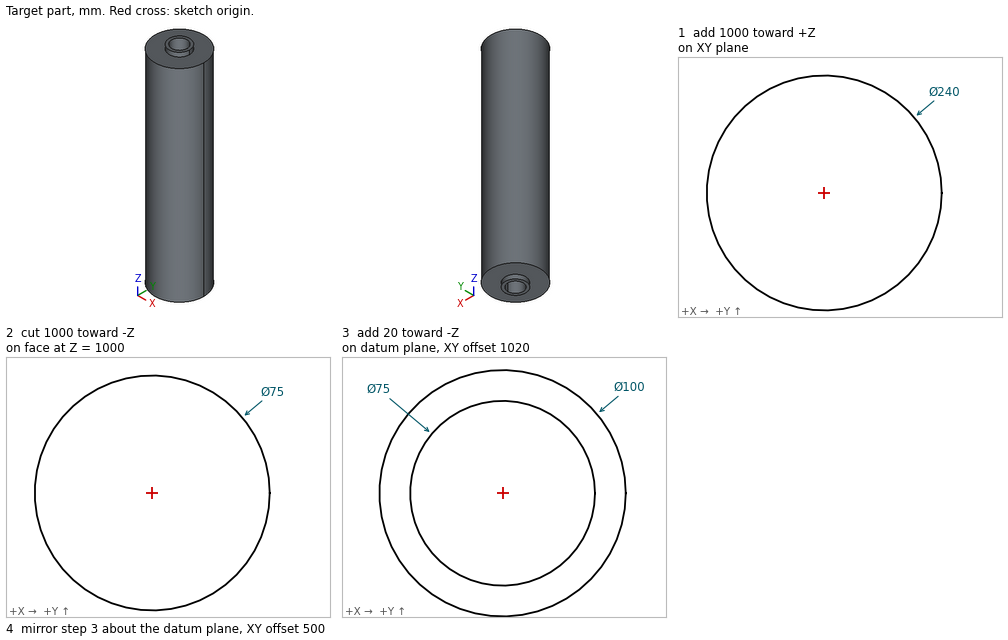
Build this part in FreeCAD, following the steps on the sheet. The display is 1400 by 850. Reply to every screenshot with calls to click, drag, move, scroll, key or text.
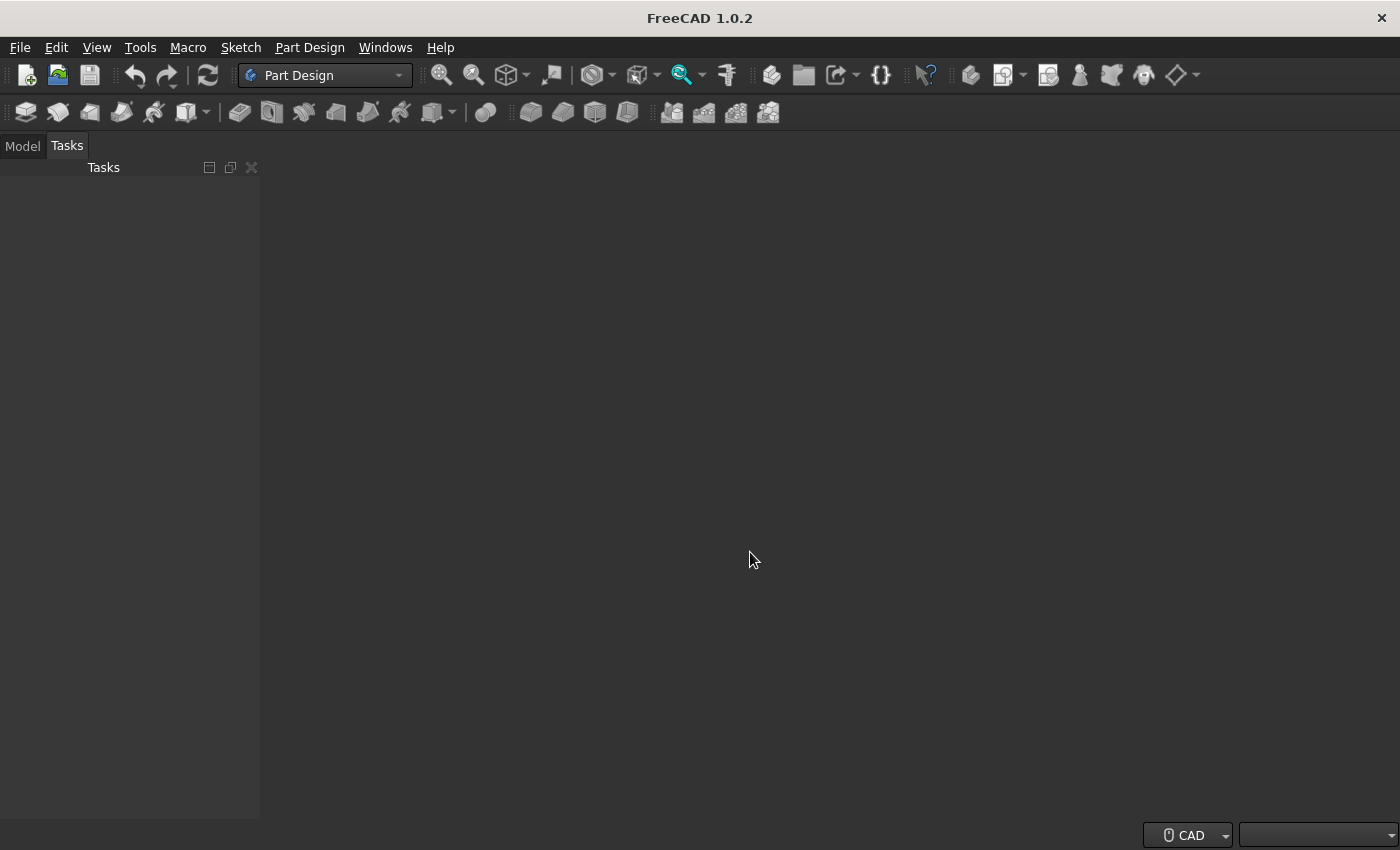
click(26, 76)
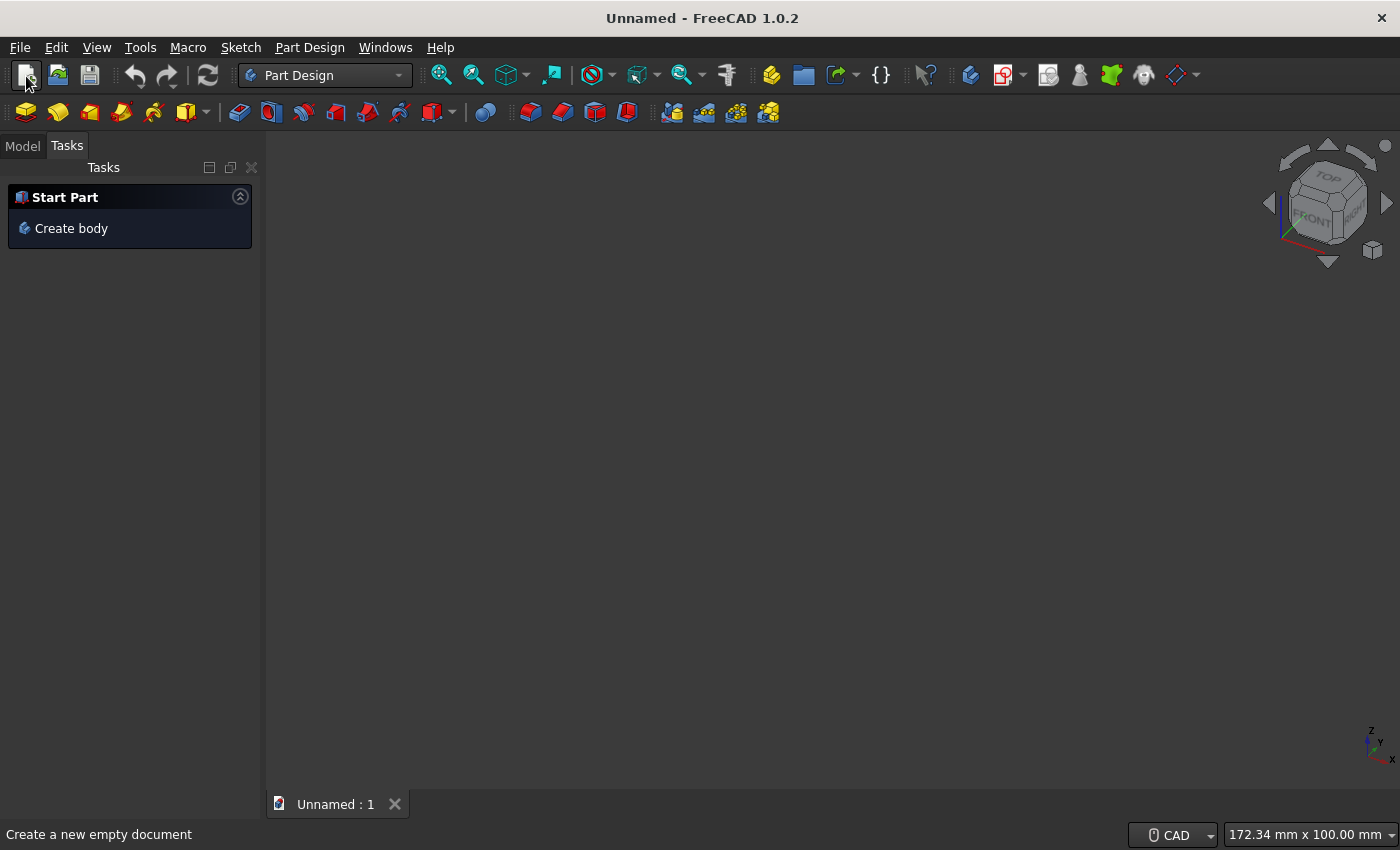
click(1004, 76)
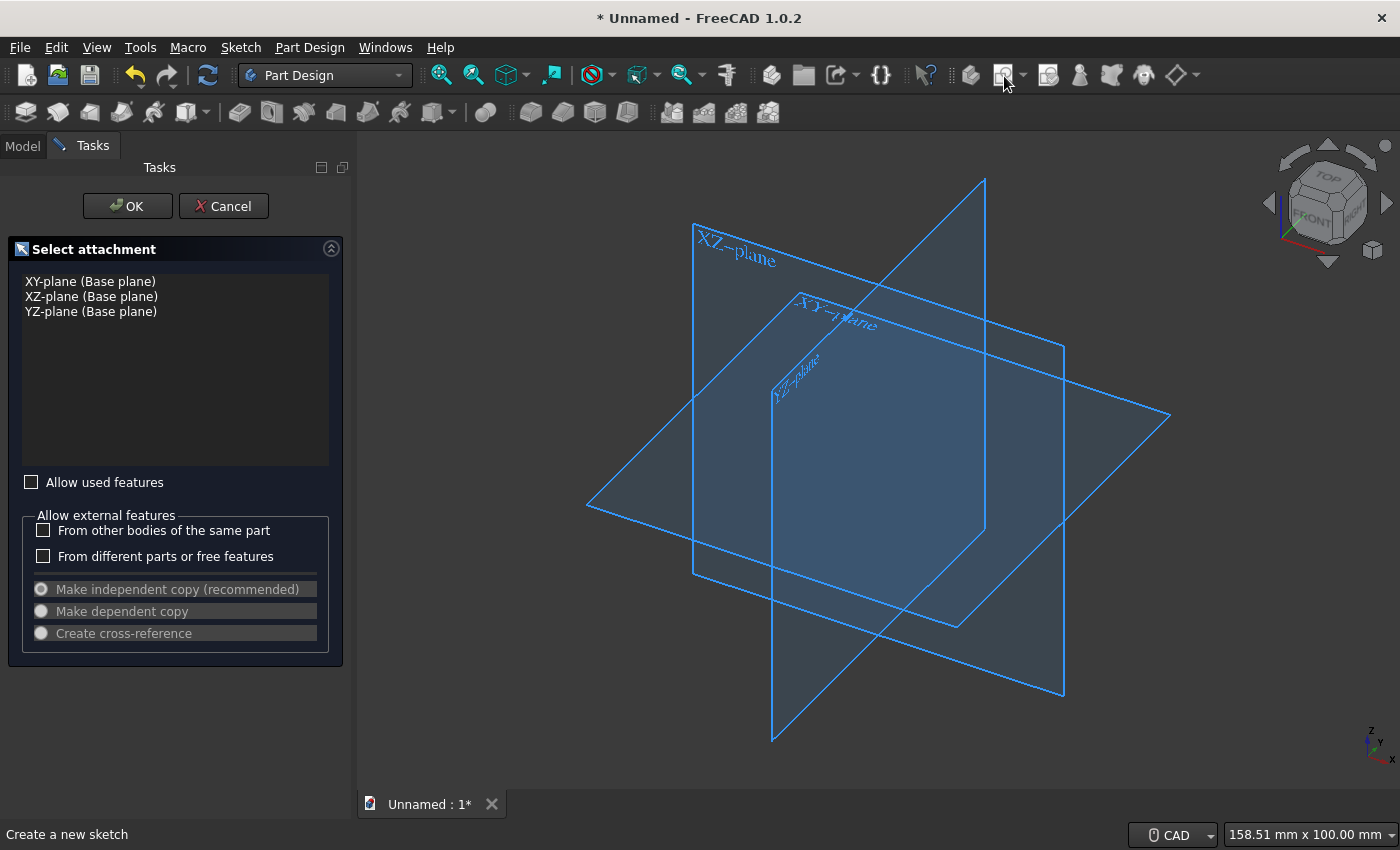
click(82, 282)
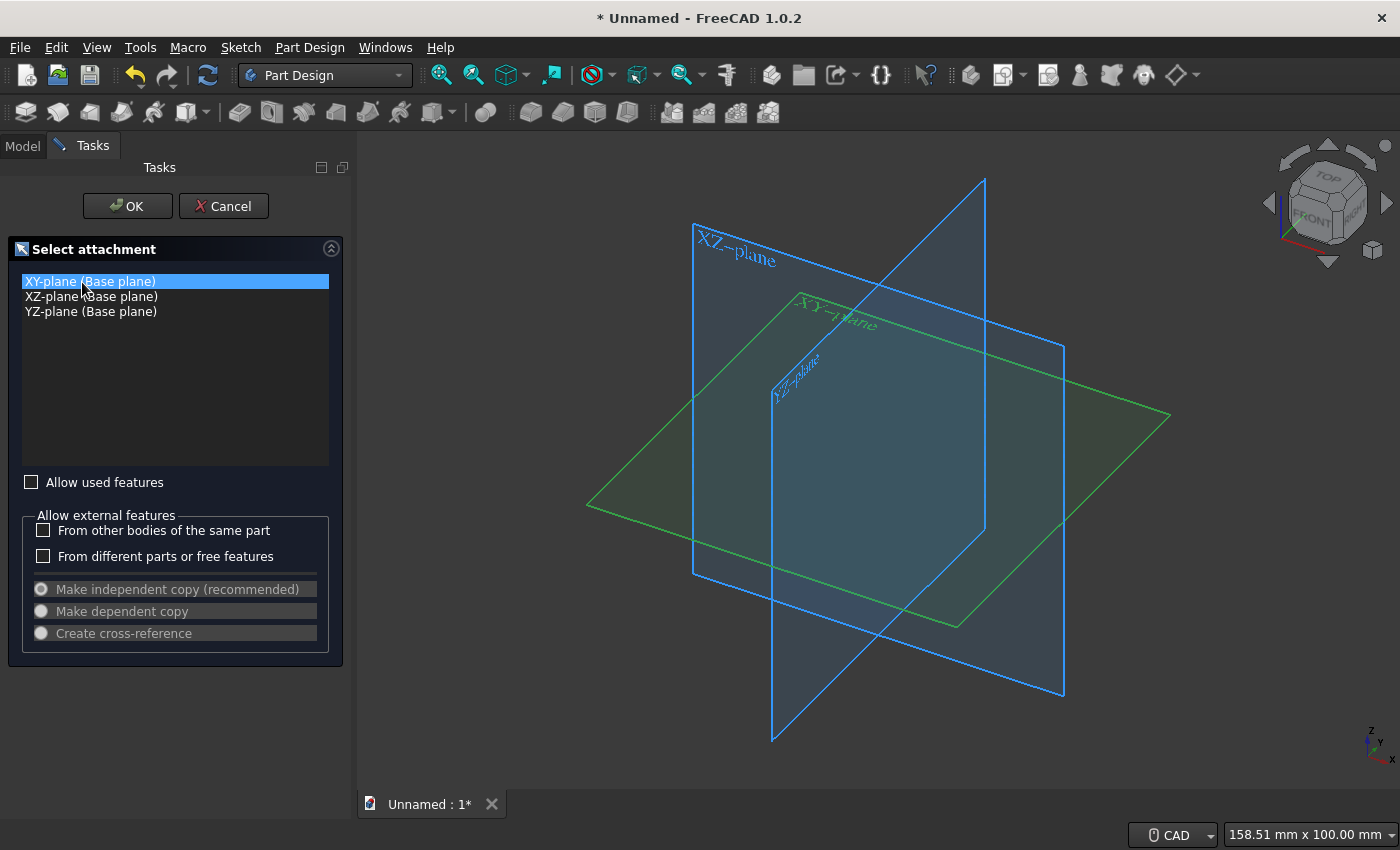
click(128, 206)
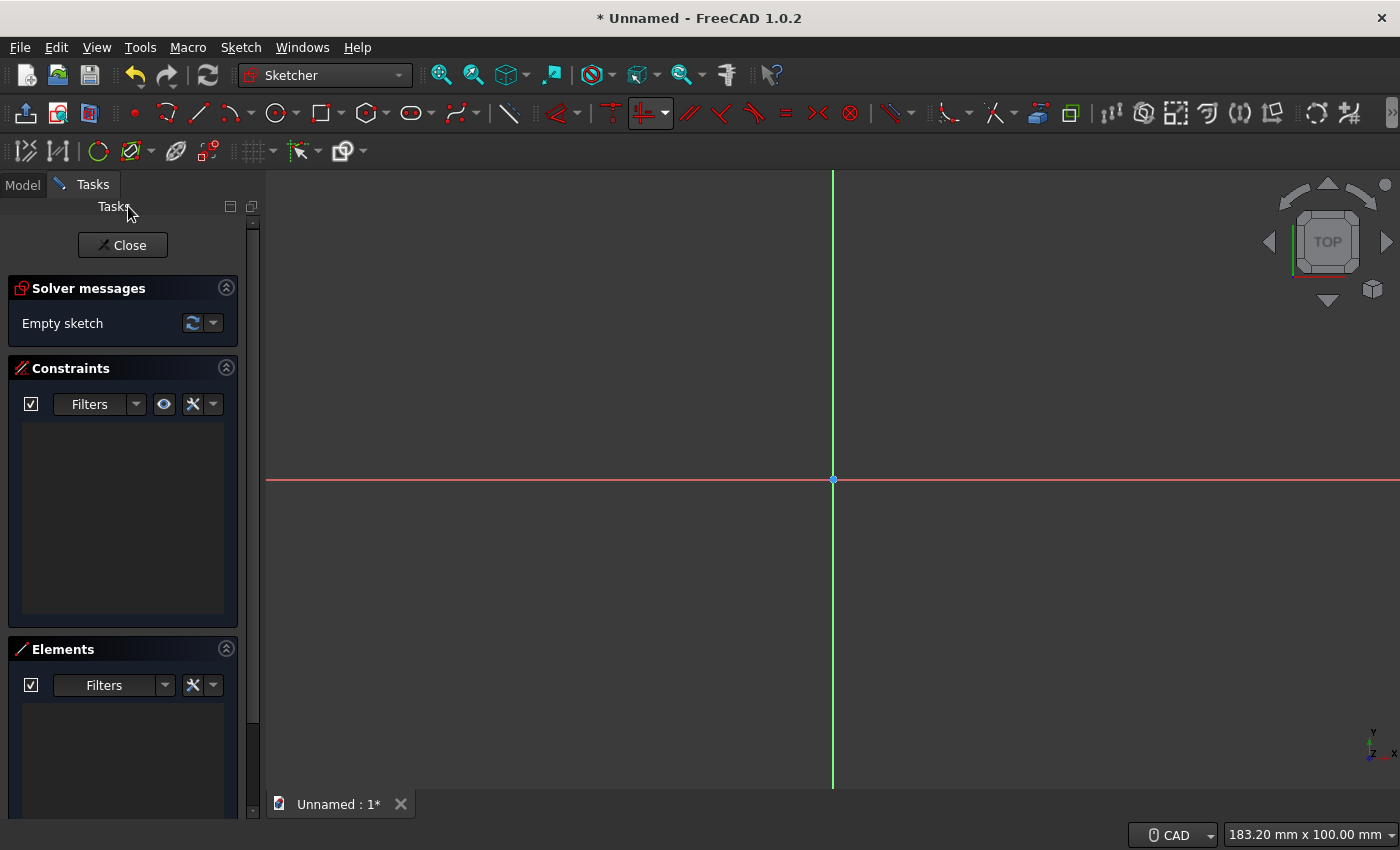
scroll(742, 480, down, 7)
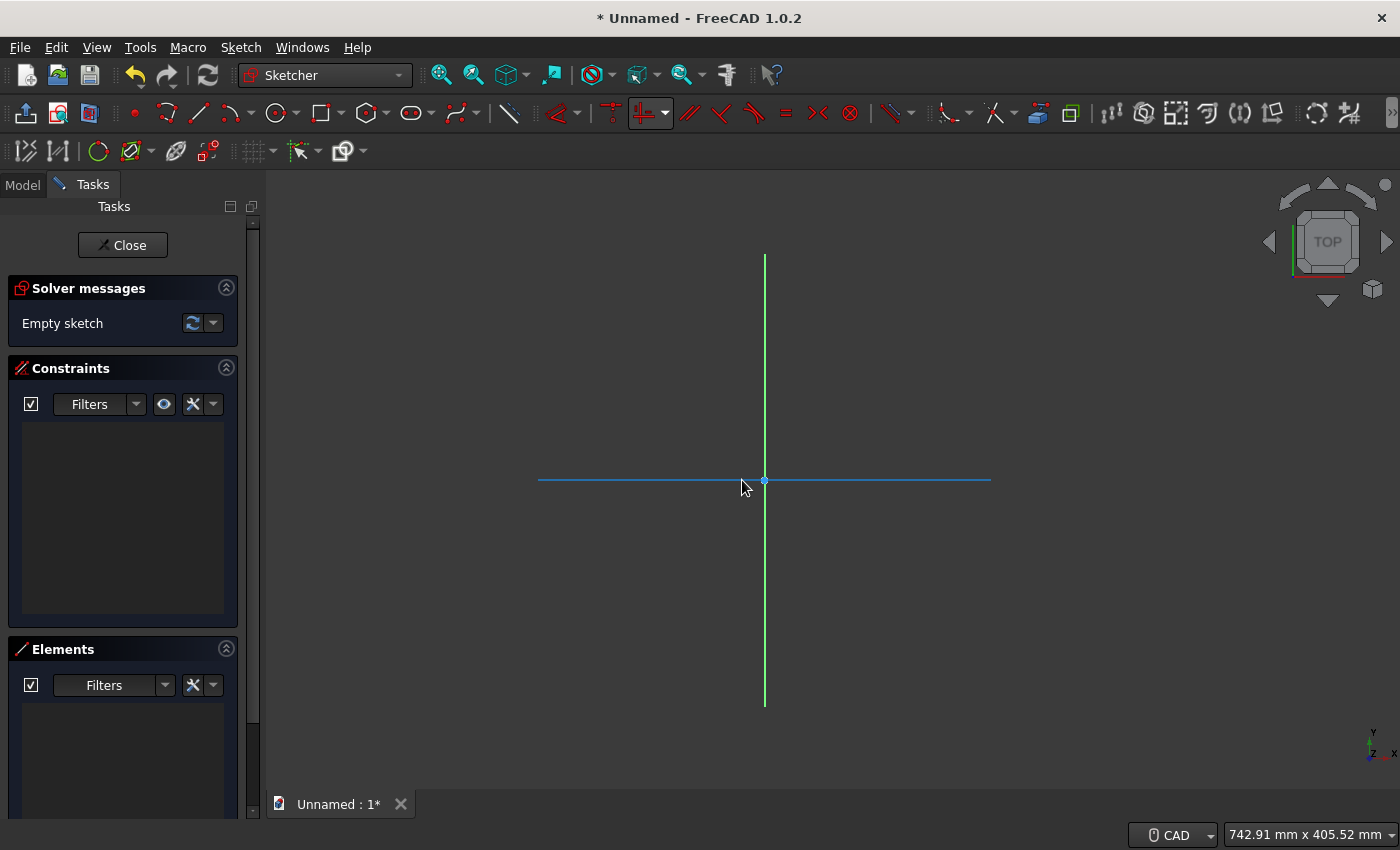
key(g)
key(c)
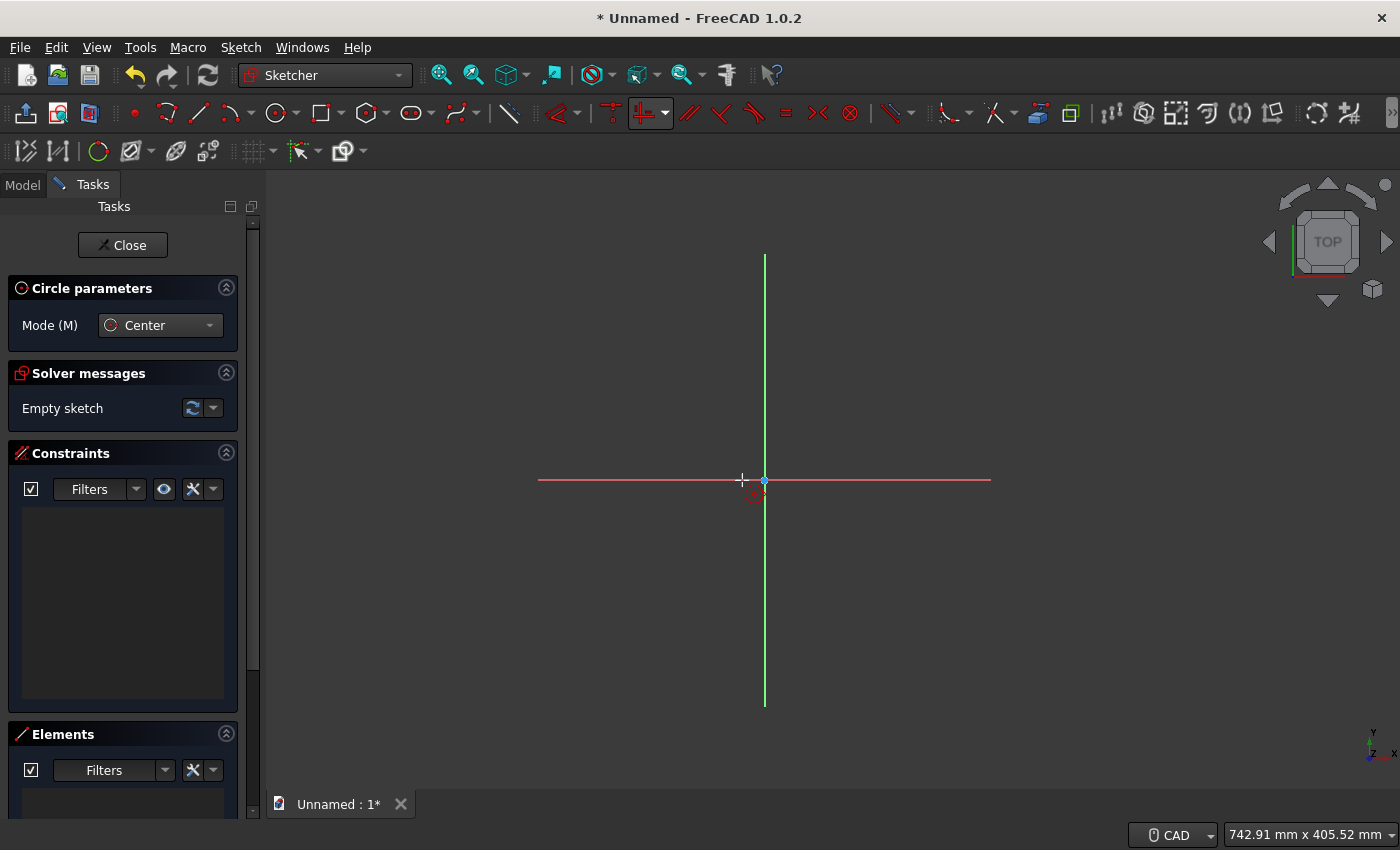
click(765, 480)
click(894, 351)
key(Escape)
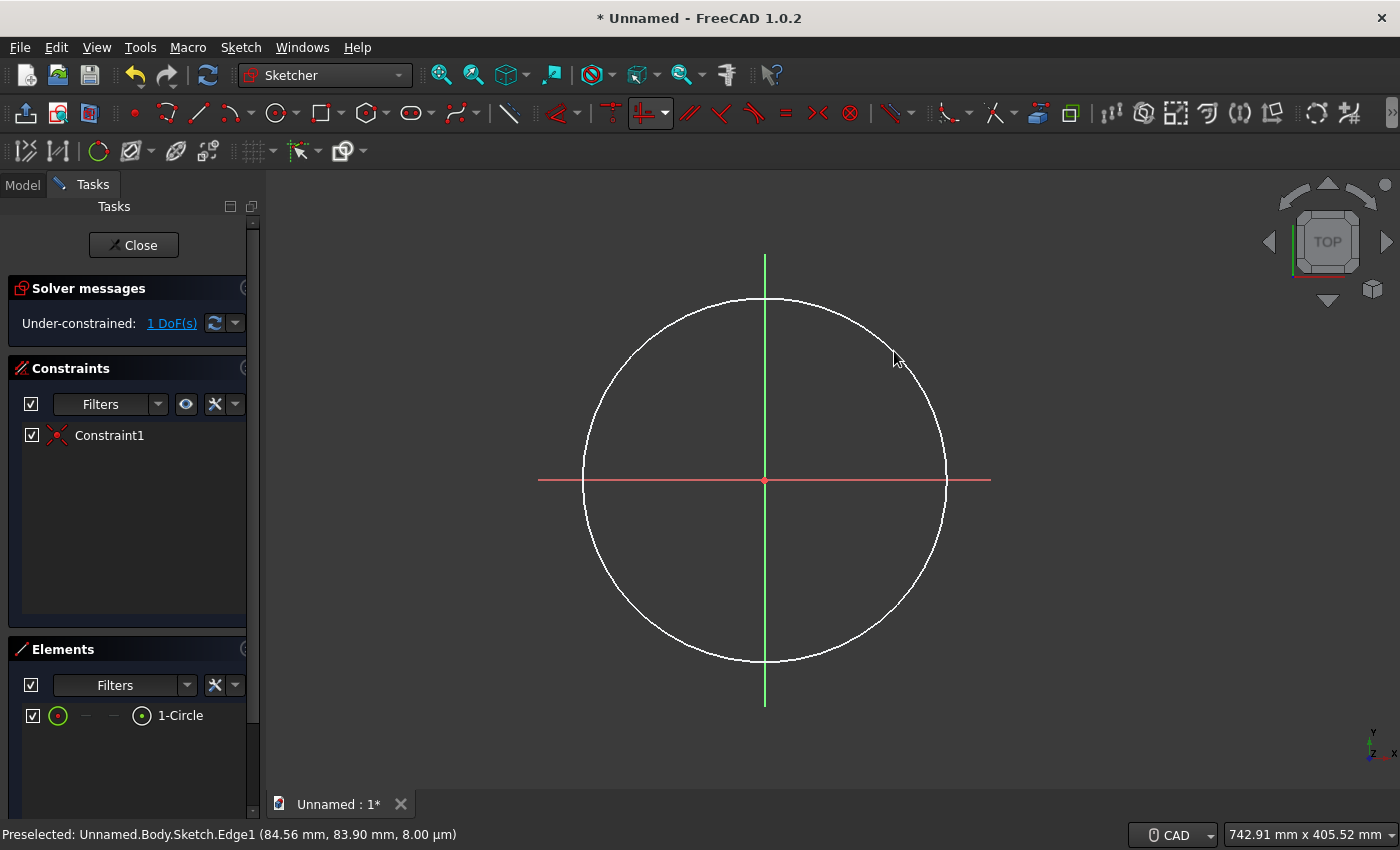
click(556, 114)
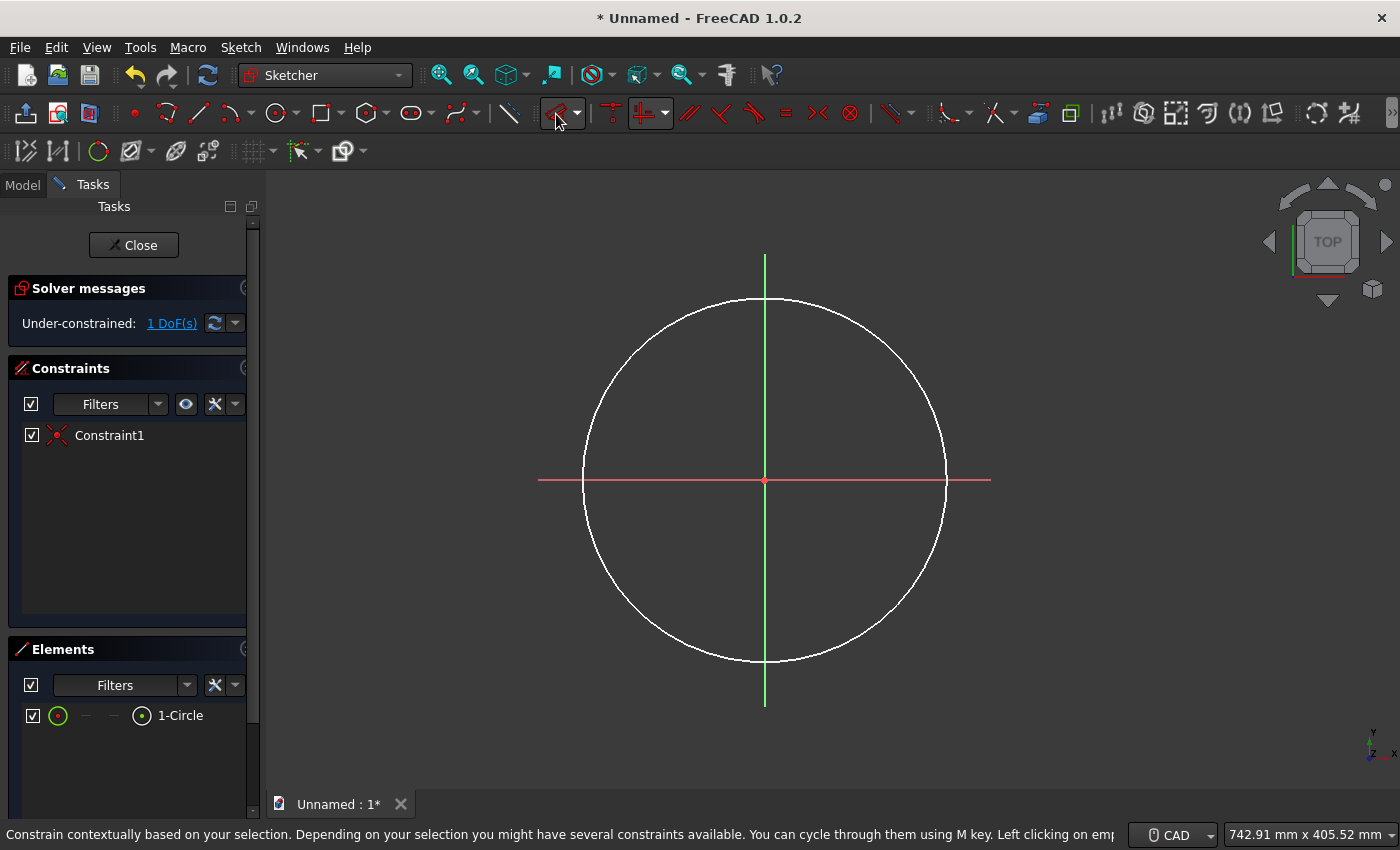
click(893, 351)
click(916, 328)